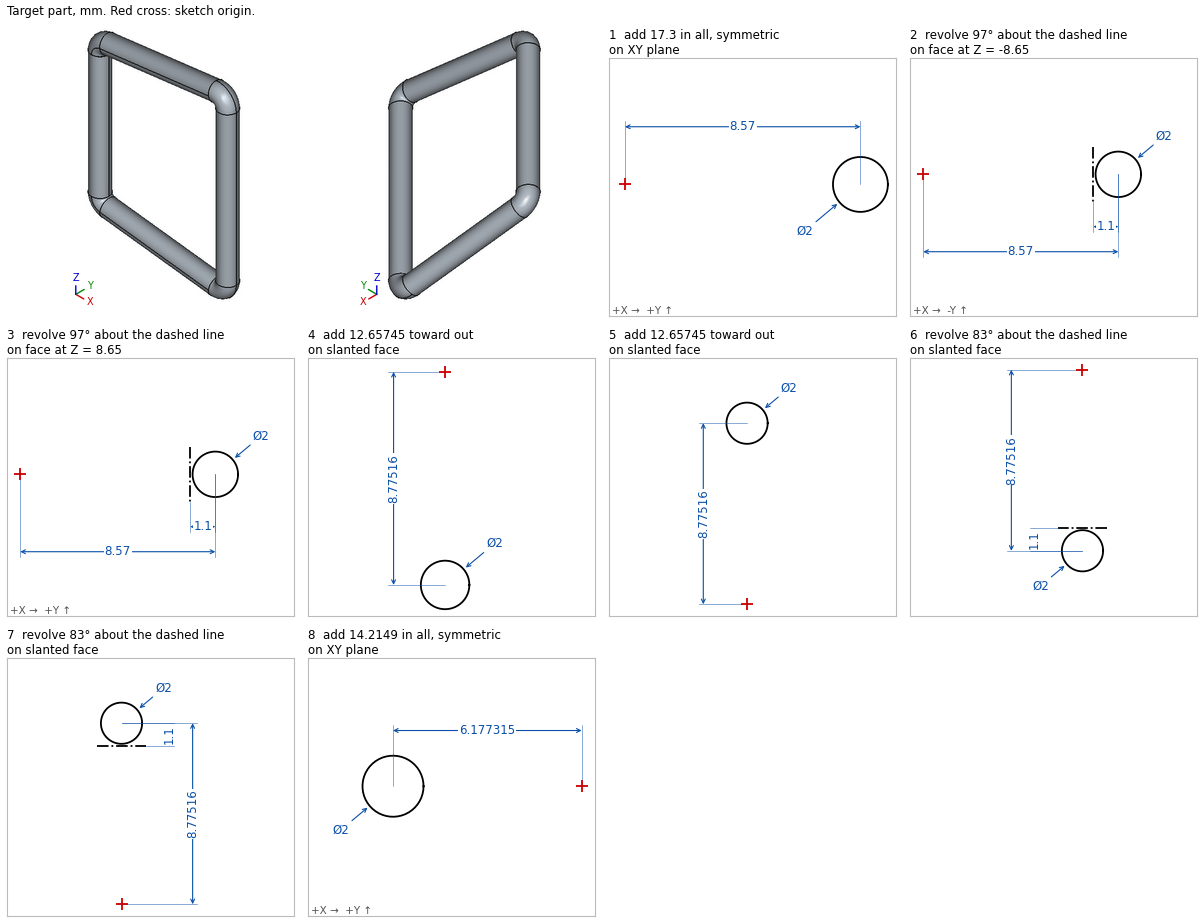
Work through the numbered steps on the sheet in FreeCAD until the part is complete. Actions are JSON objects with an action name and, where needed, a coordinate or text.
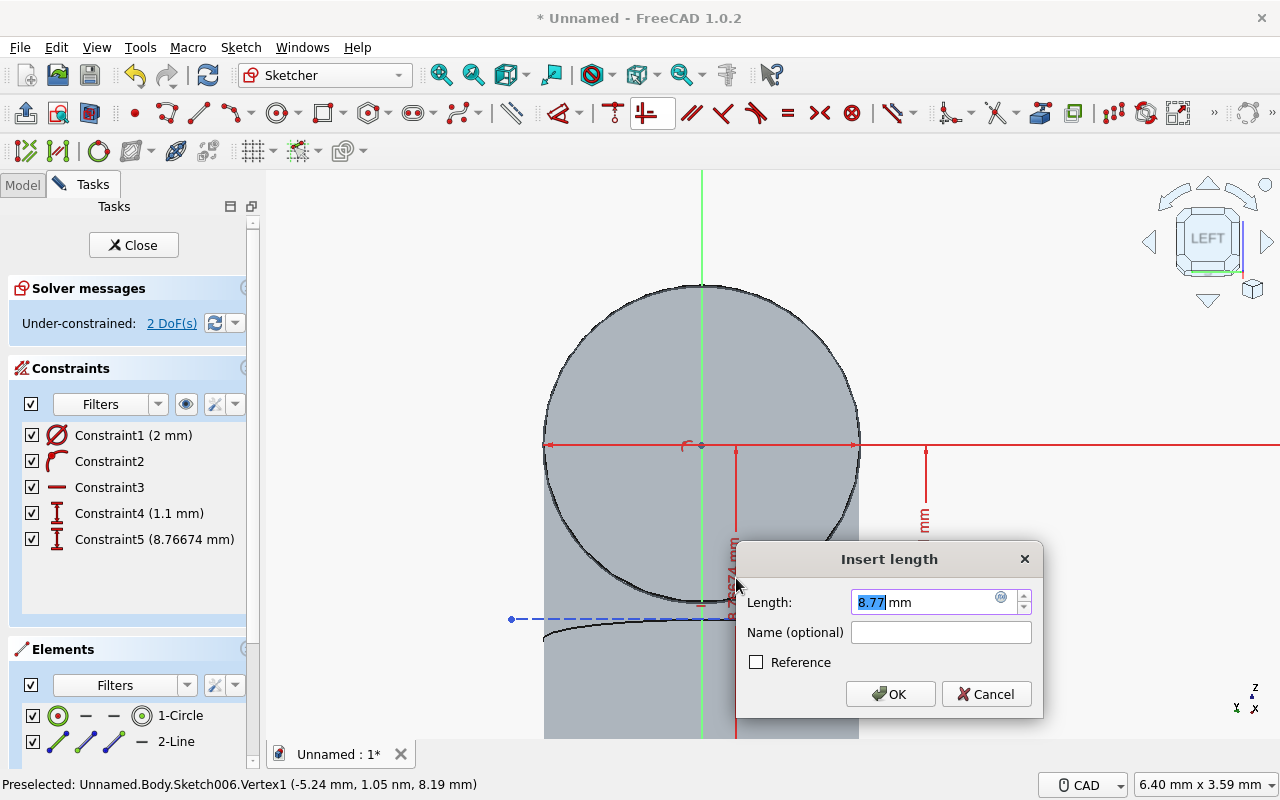
{"action": "type", "text": "8.77516"}
{"action": "key", "text": "Return"}
{"action": "key", "text": "Escape"}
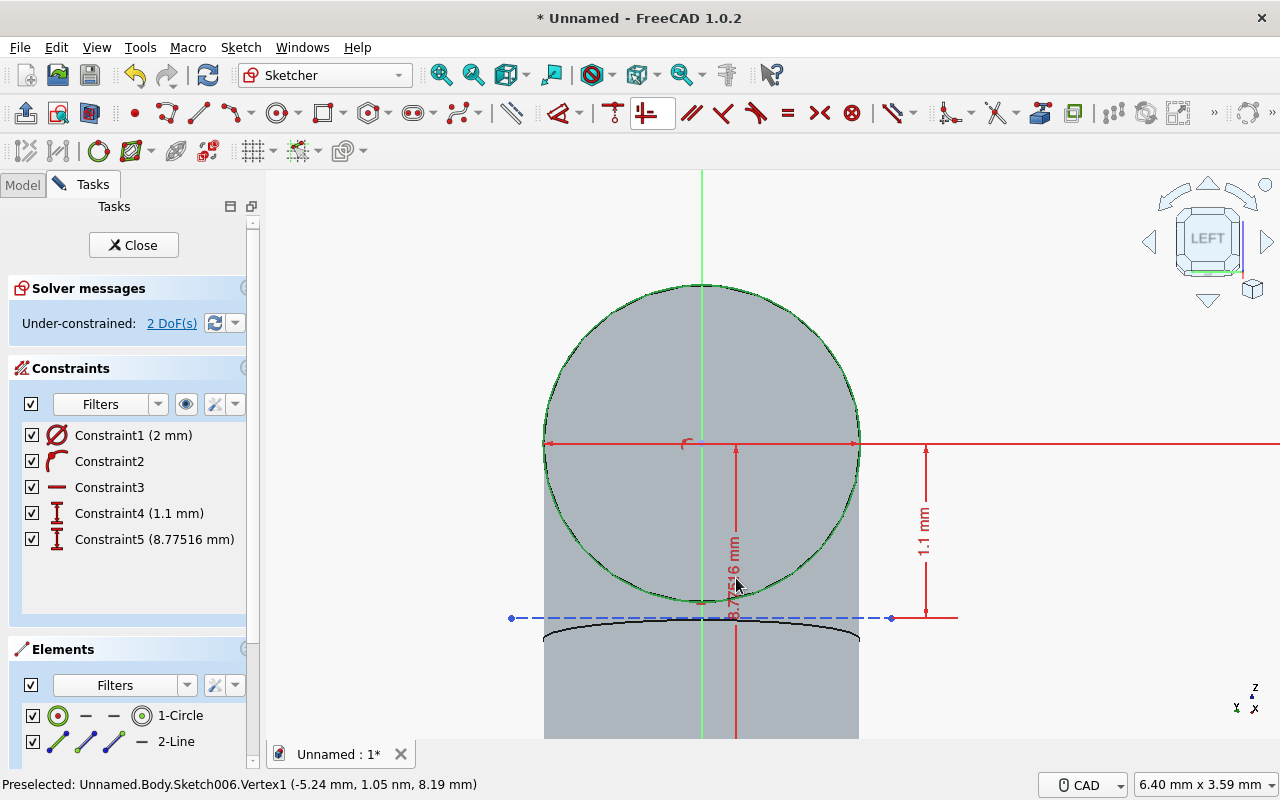
{"action": "left_click", "coordinate": [134, 245]}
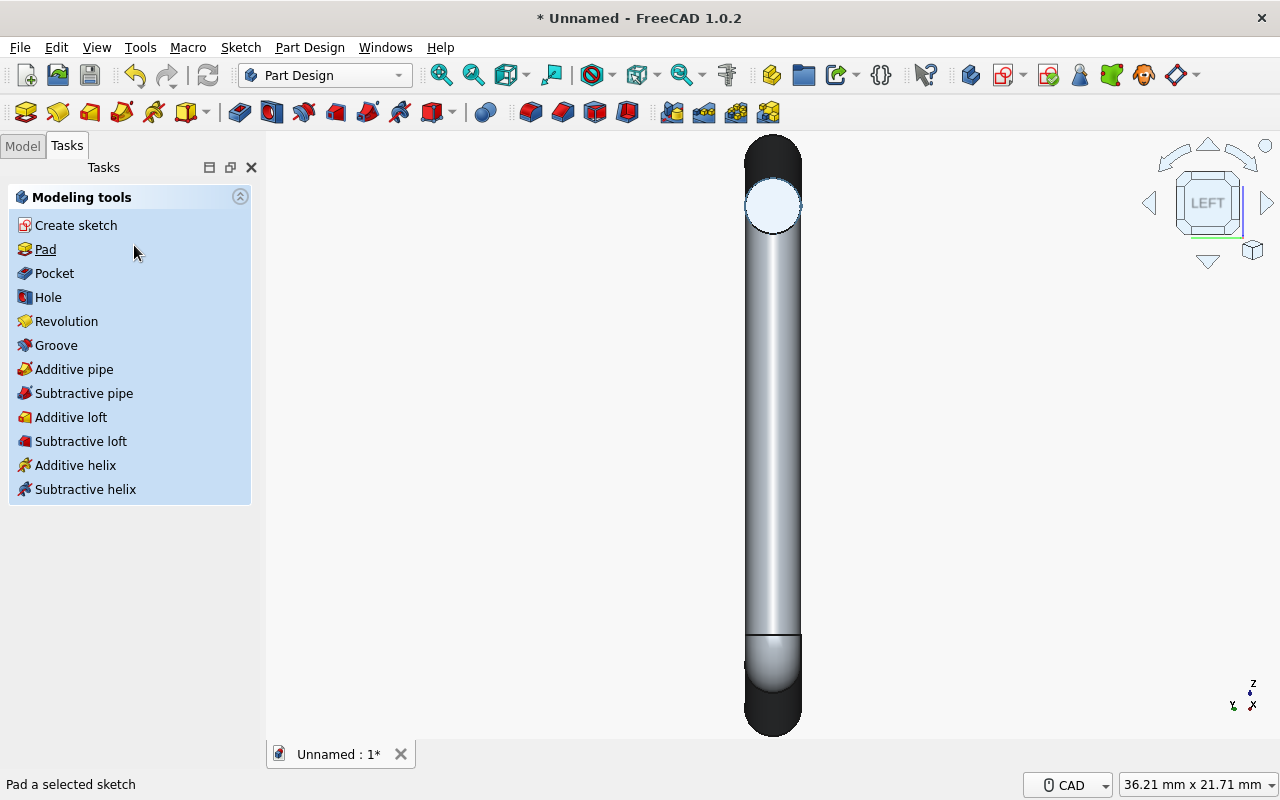
{"action": "left_click", "coordinate": [58, 112]}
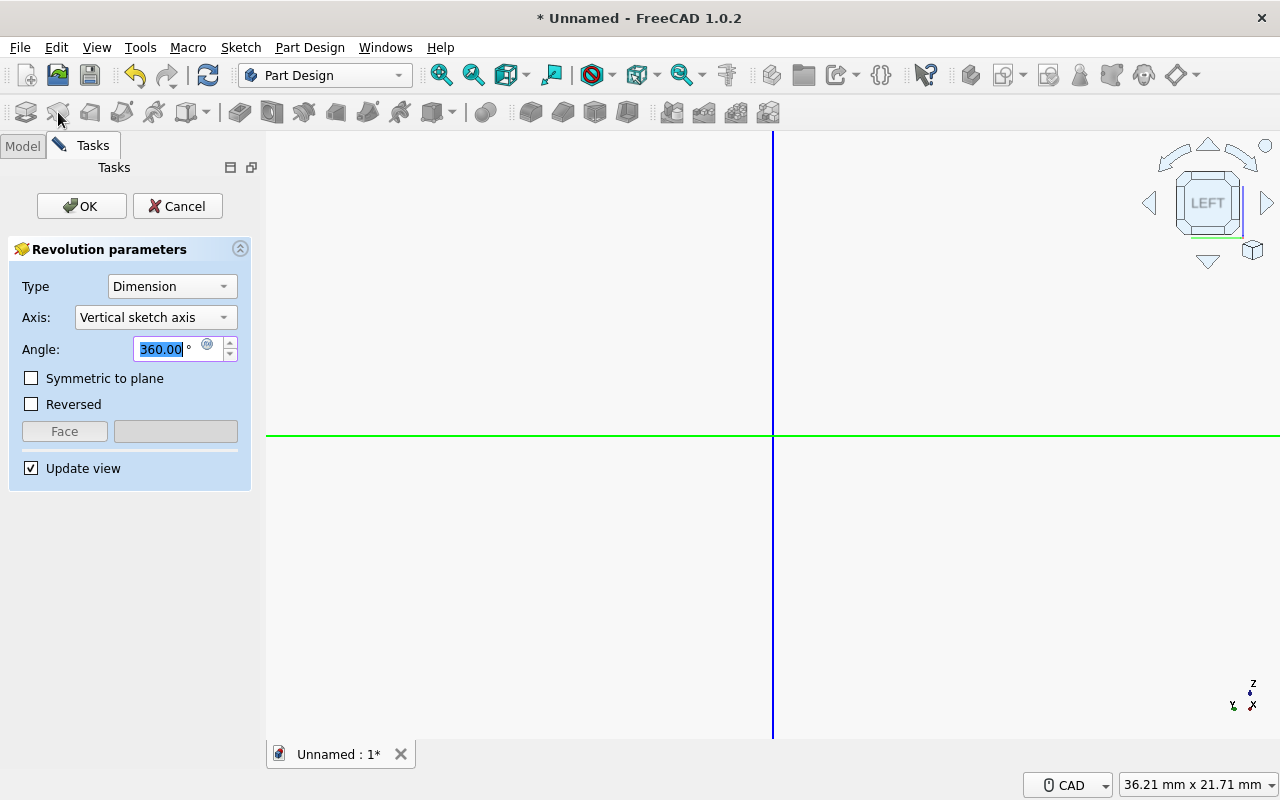
{"action": "left_click", "coordinate": [156, 318]}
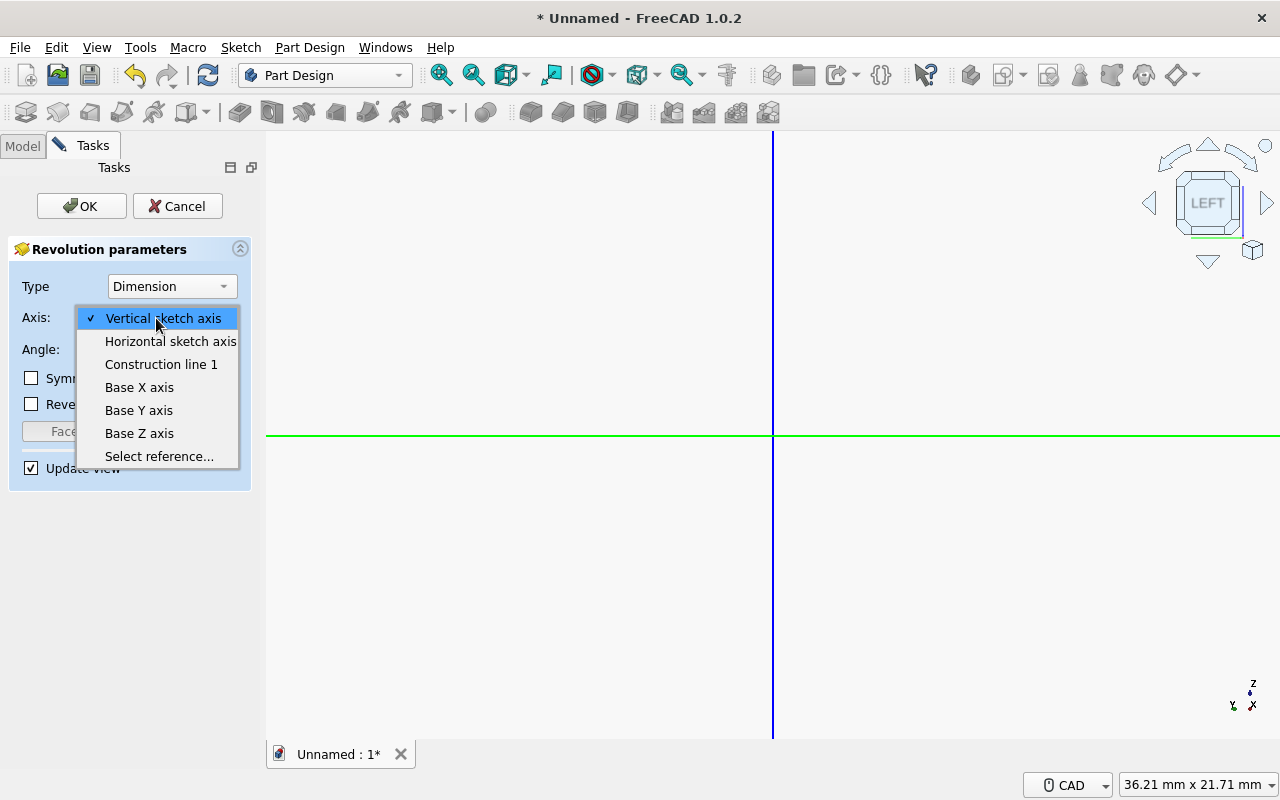
{"action": "left_click", "coordinate": [156, 364]}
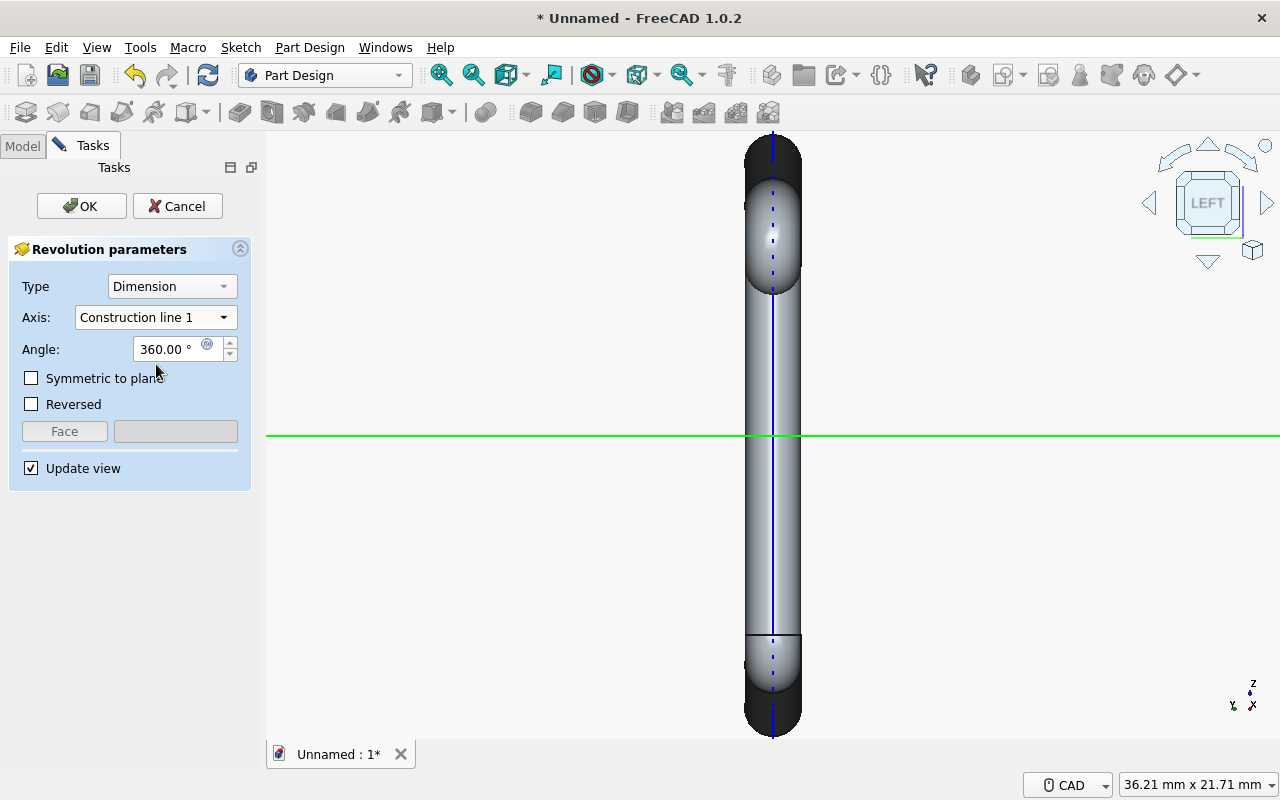
{"action": "triple_click", "coordinate": [178, 349]}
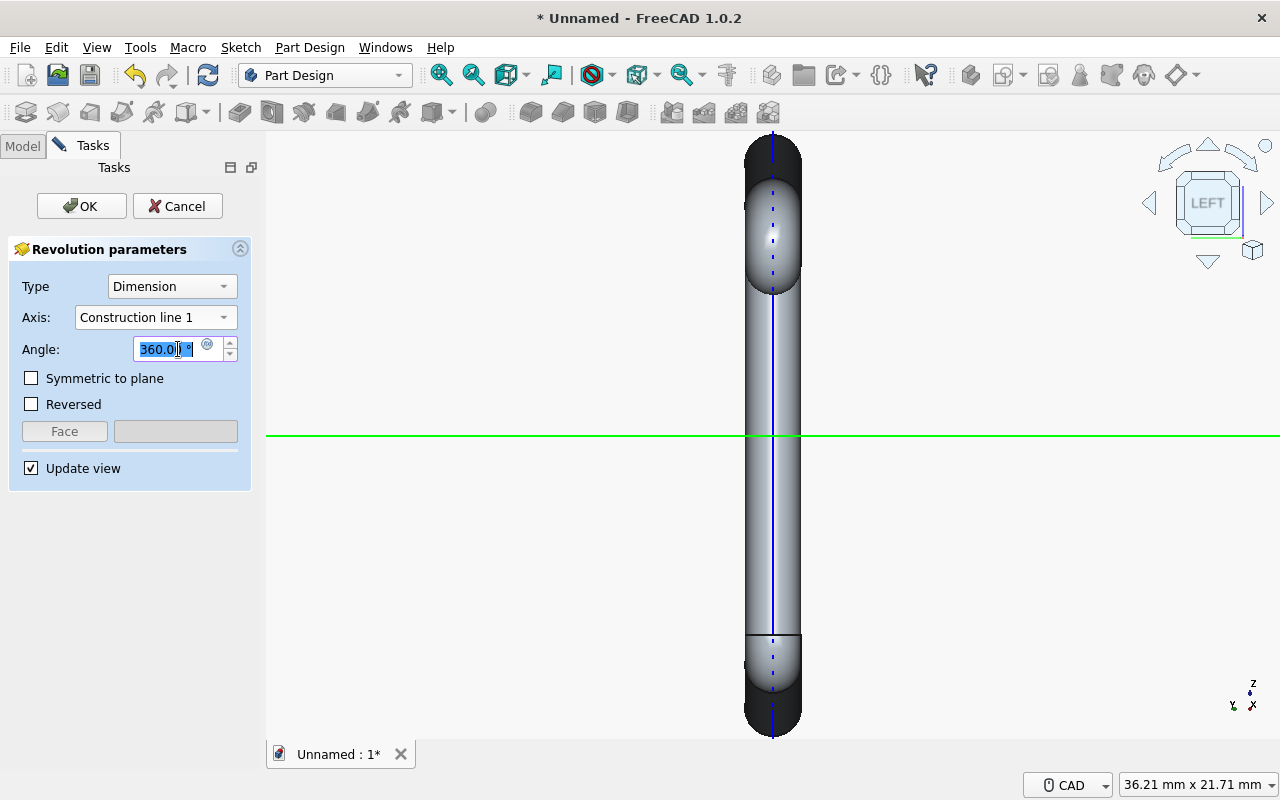
{"action": "type", "text": "83"}
{"action": "key", "text": "Tab"}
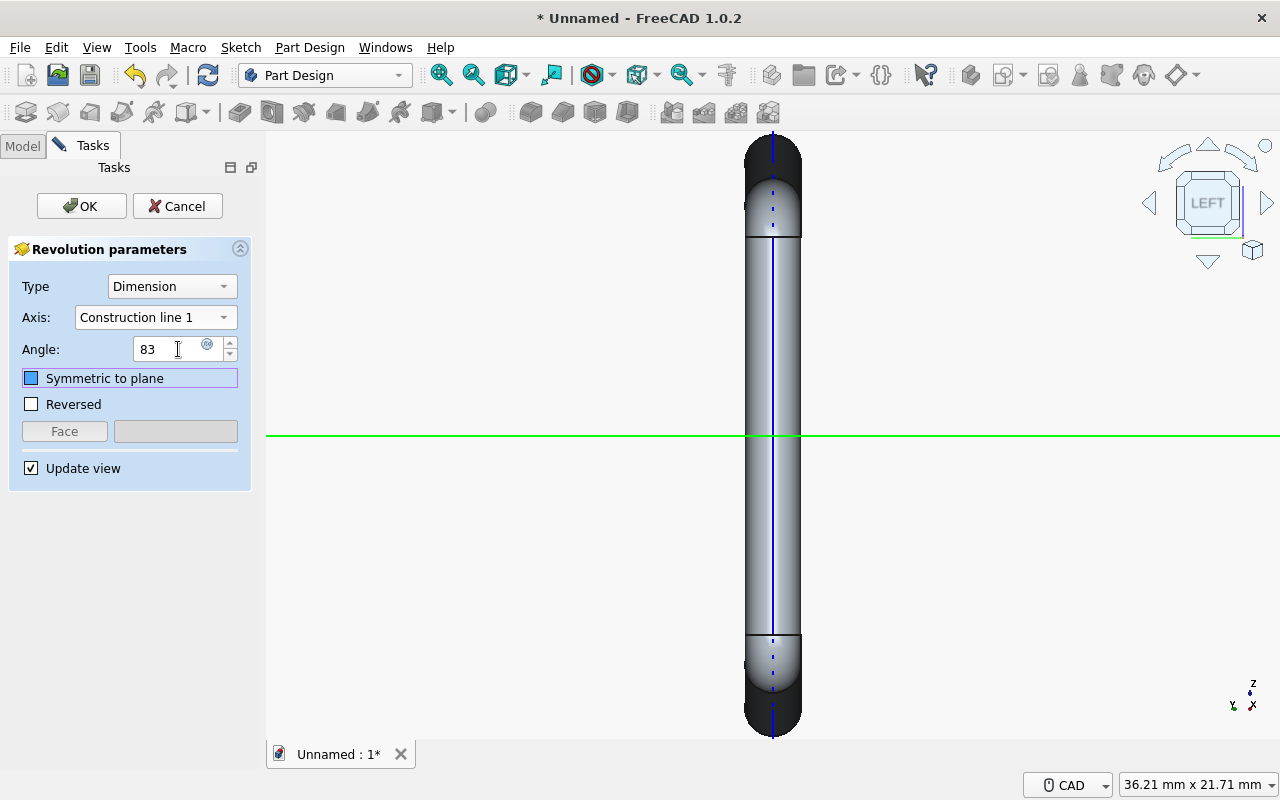
{"action": "left_click", "coordinate": [82, 206]}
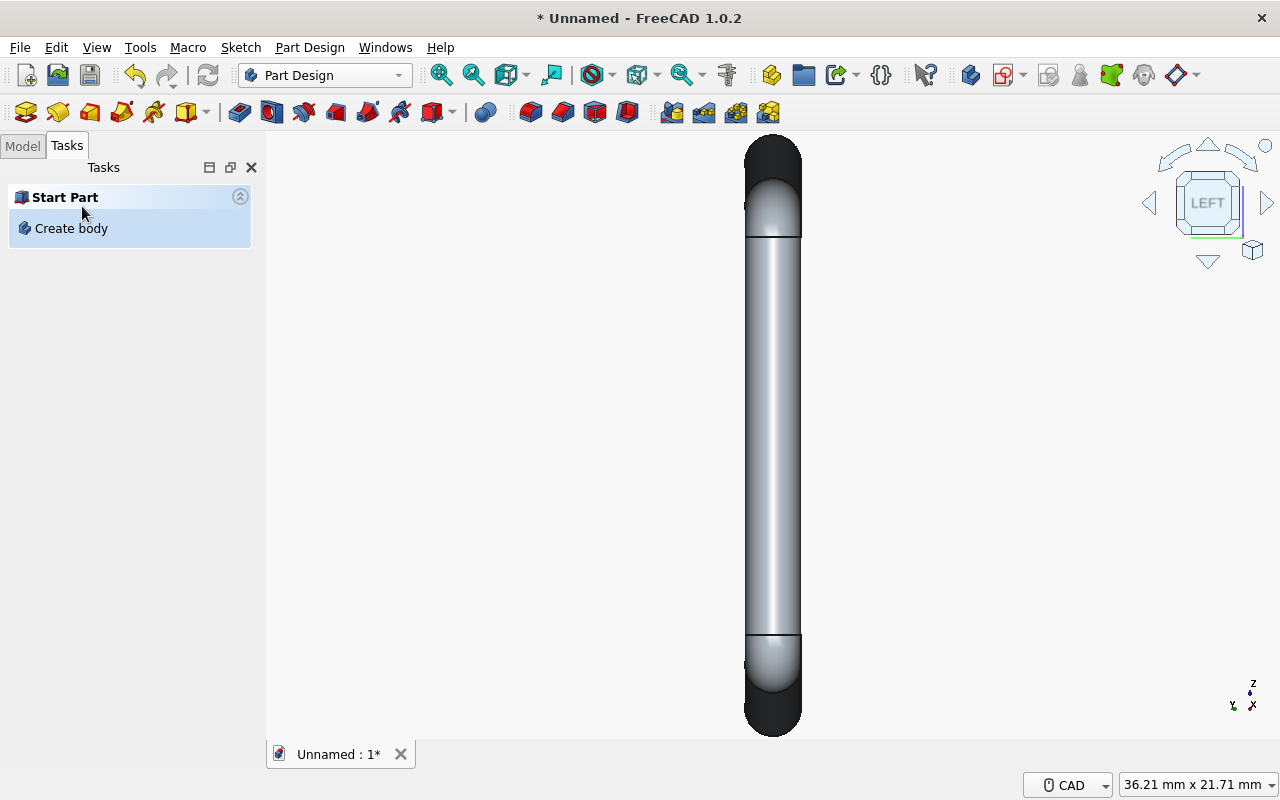
{"action": "left_click", "coordinate": [1004, 76]}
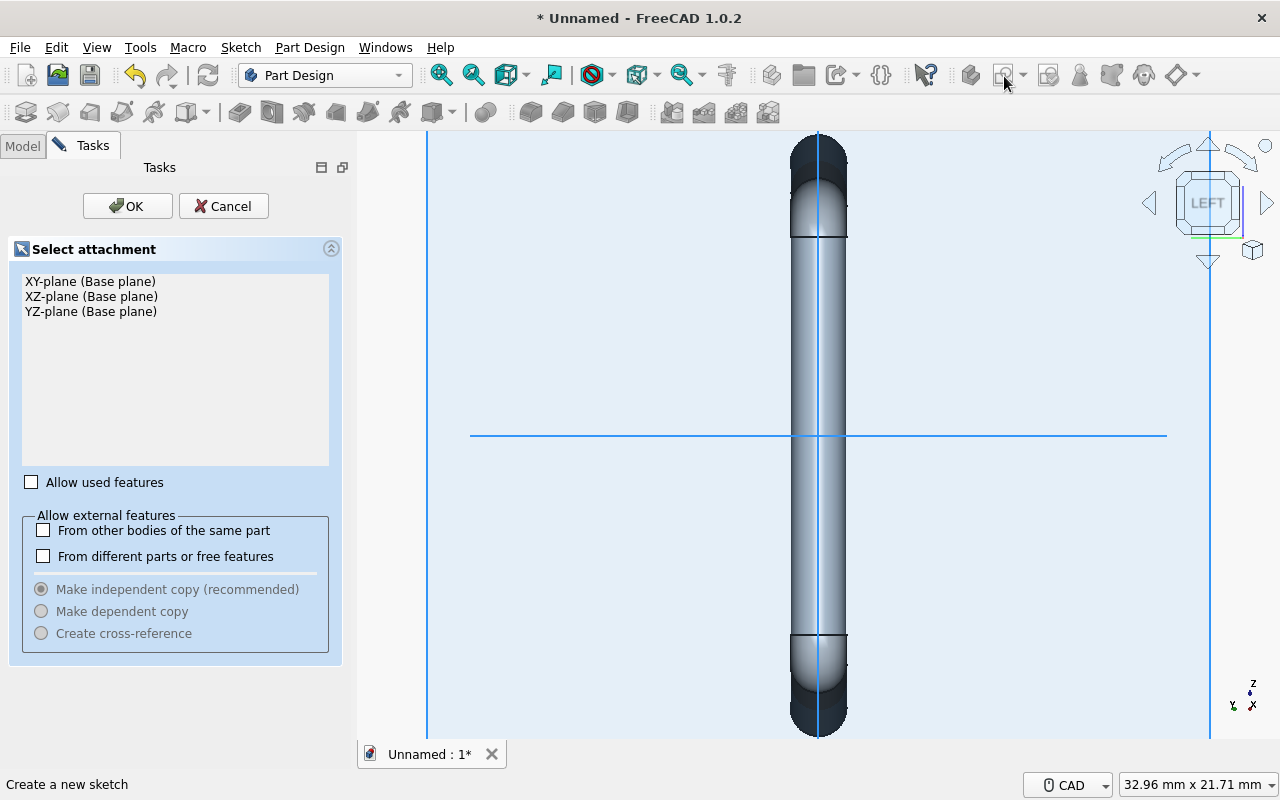
{"action": "left_click", "coordinate": [82, 282]}